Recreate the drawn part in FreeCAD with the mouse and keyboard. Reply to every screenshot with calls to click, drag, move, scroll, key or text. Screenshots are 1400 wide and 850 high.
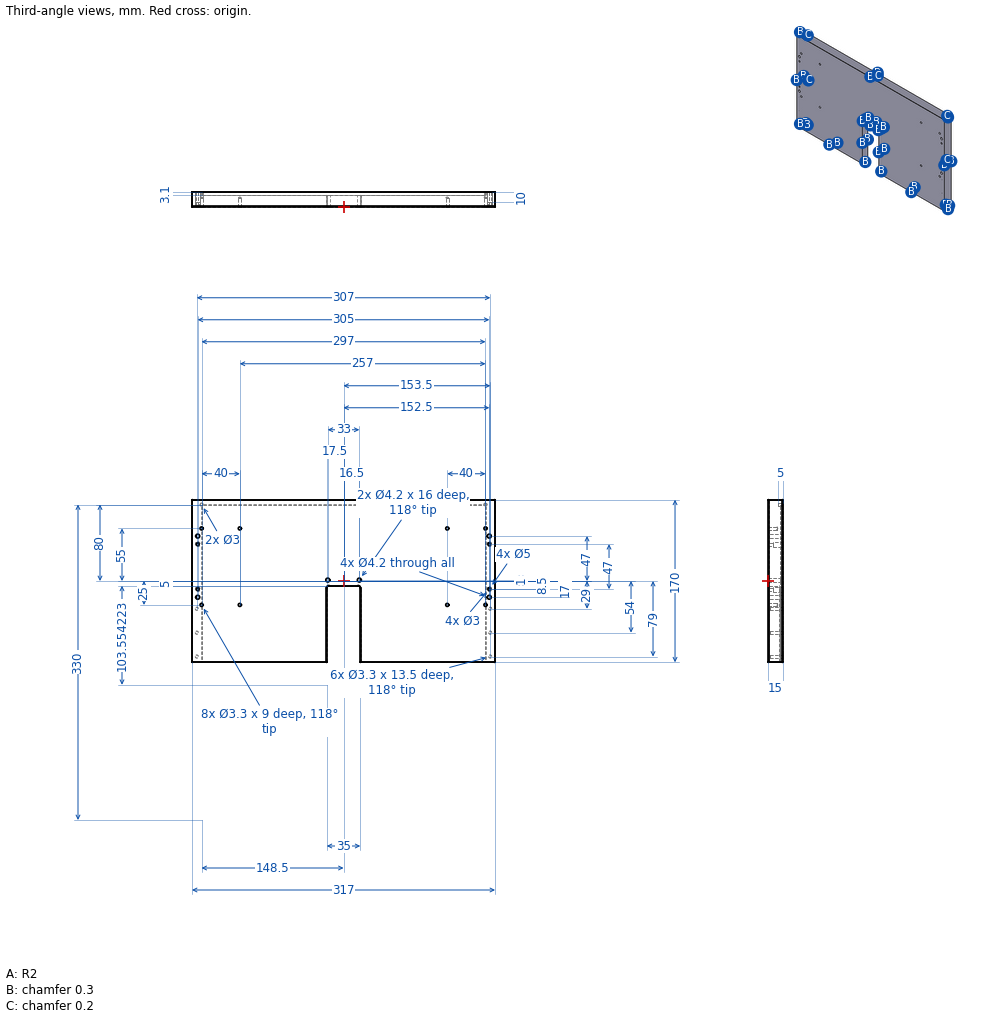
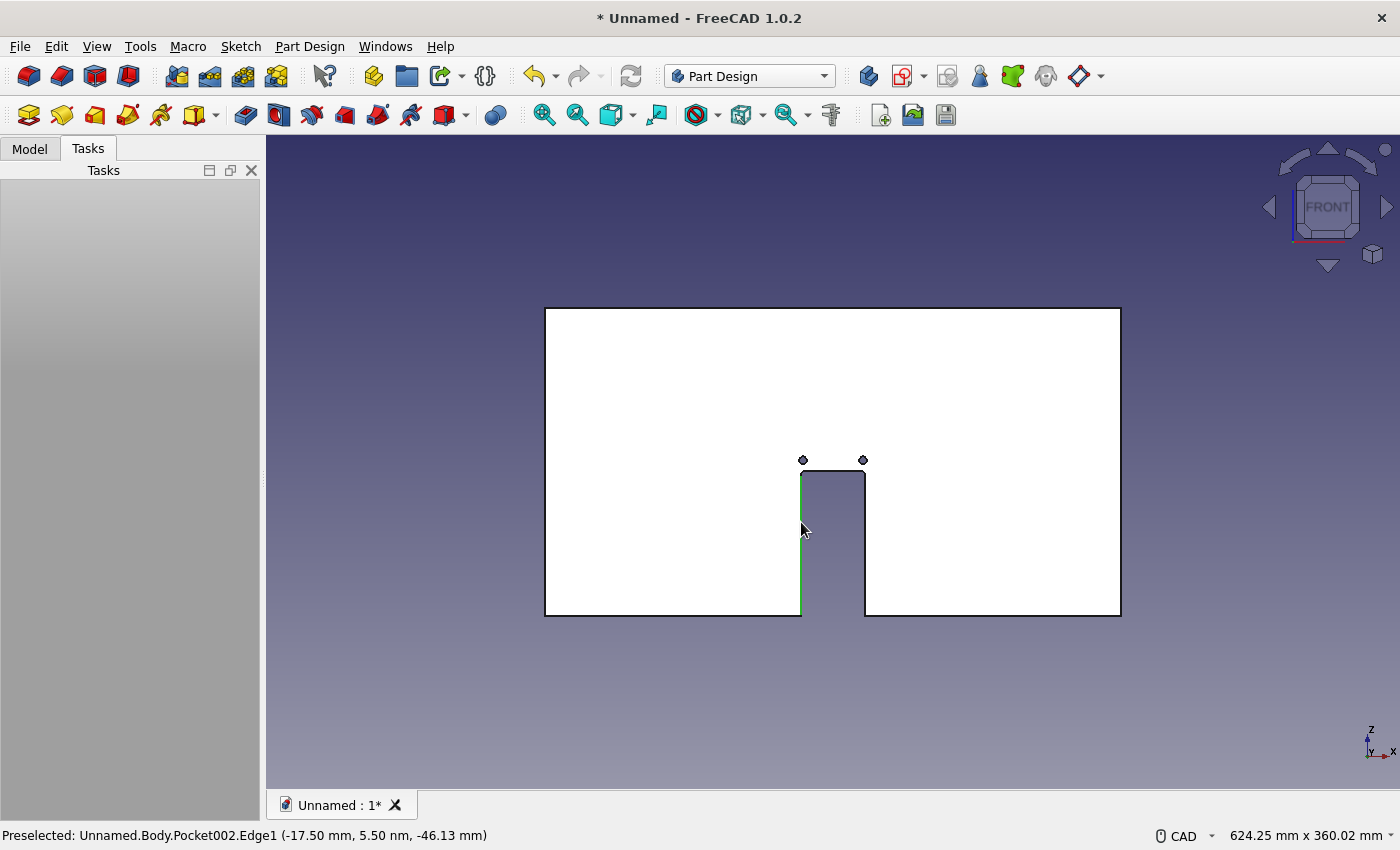
click(865, 545, ctrl)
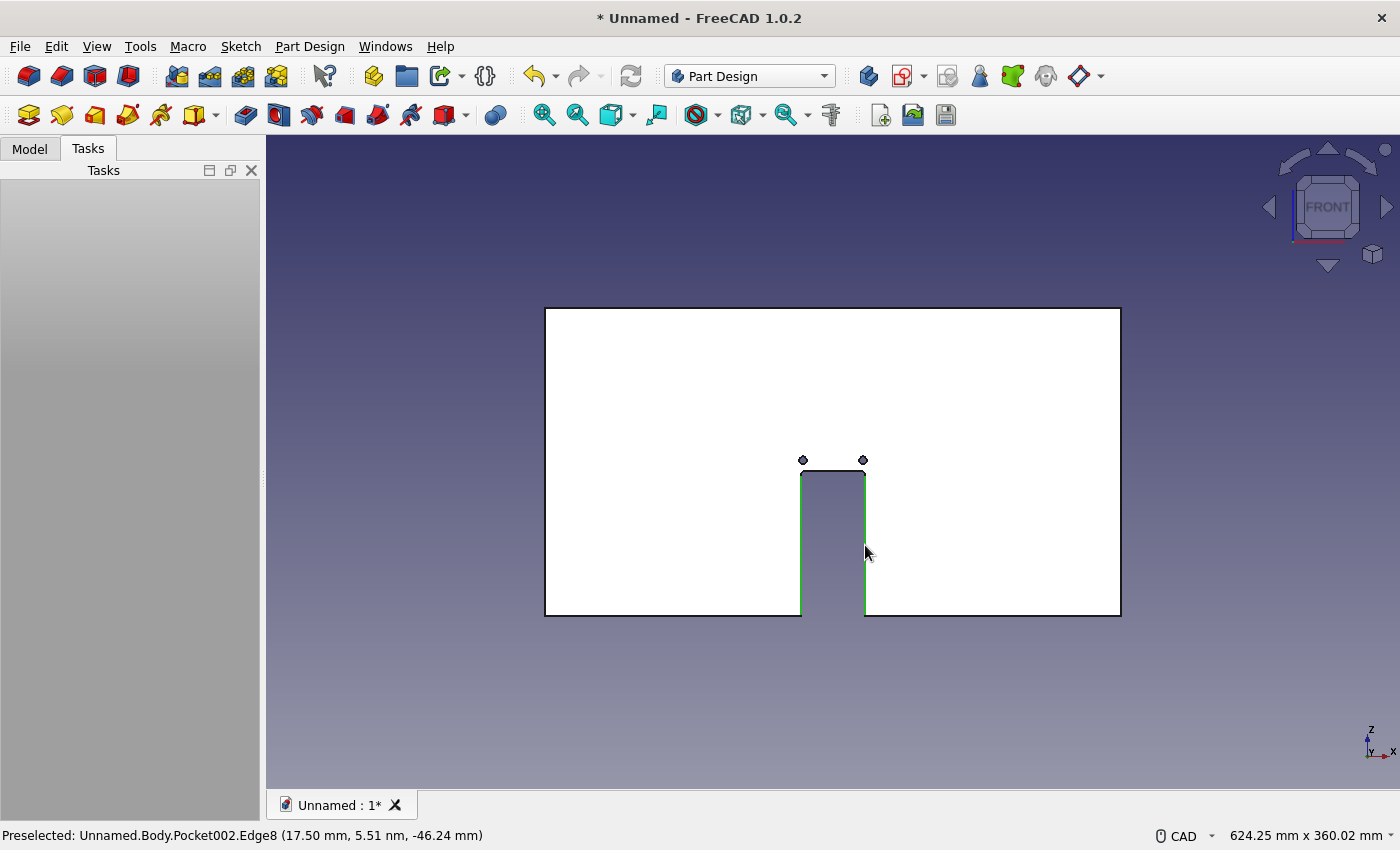
key(3)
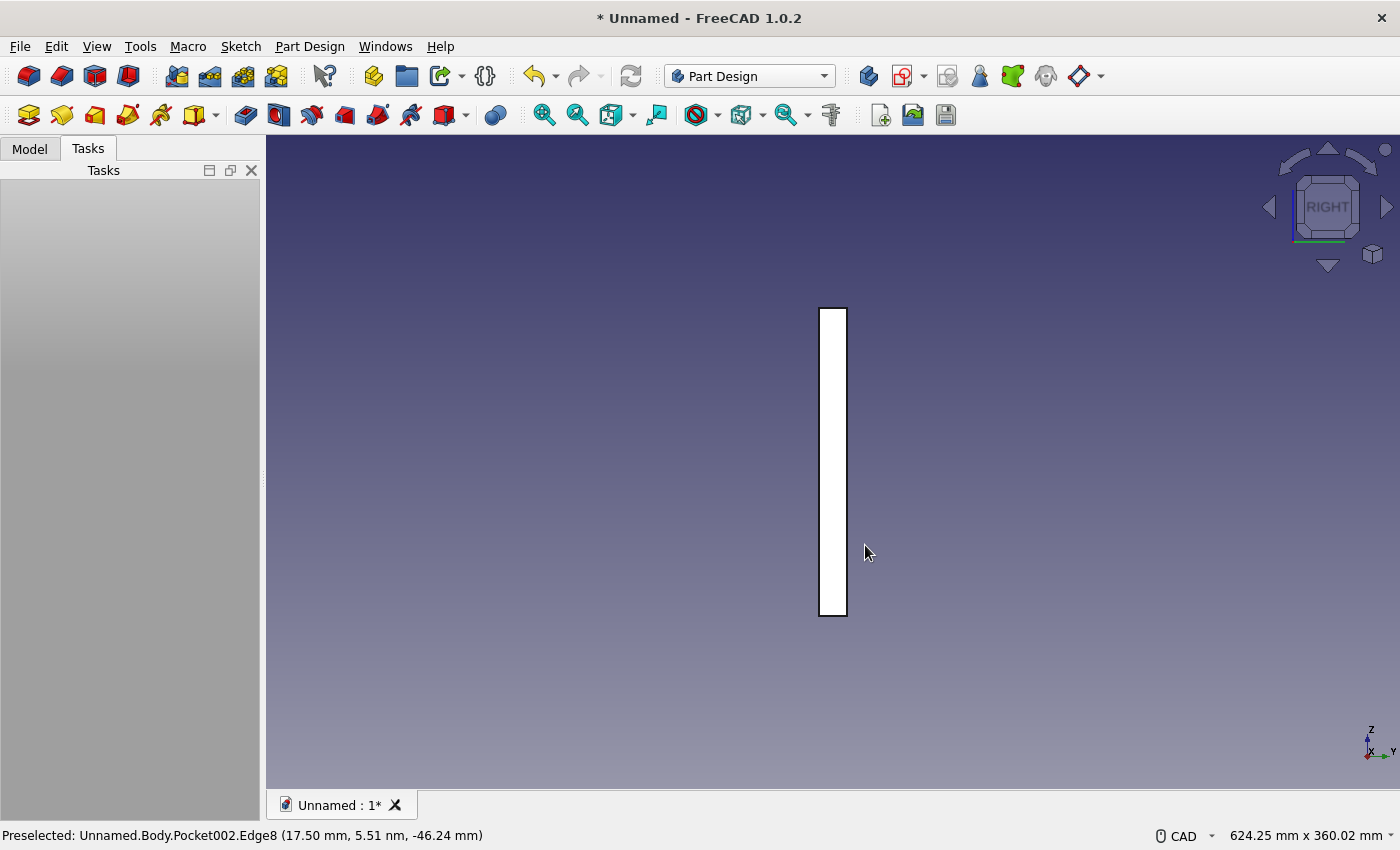
key(5)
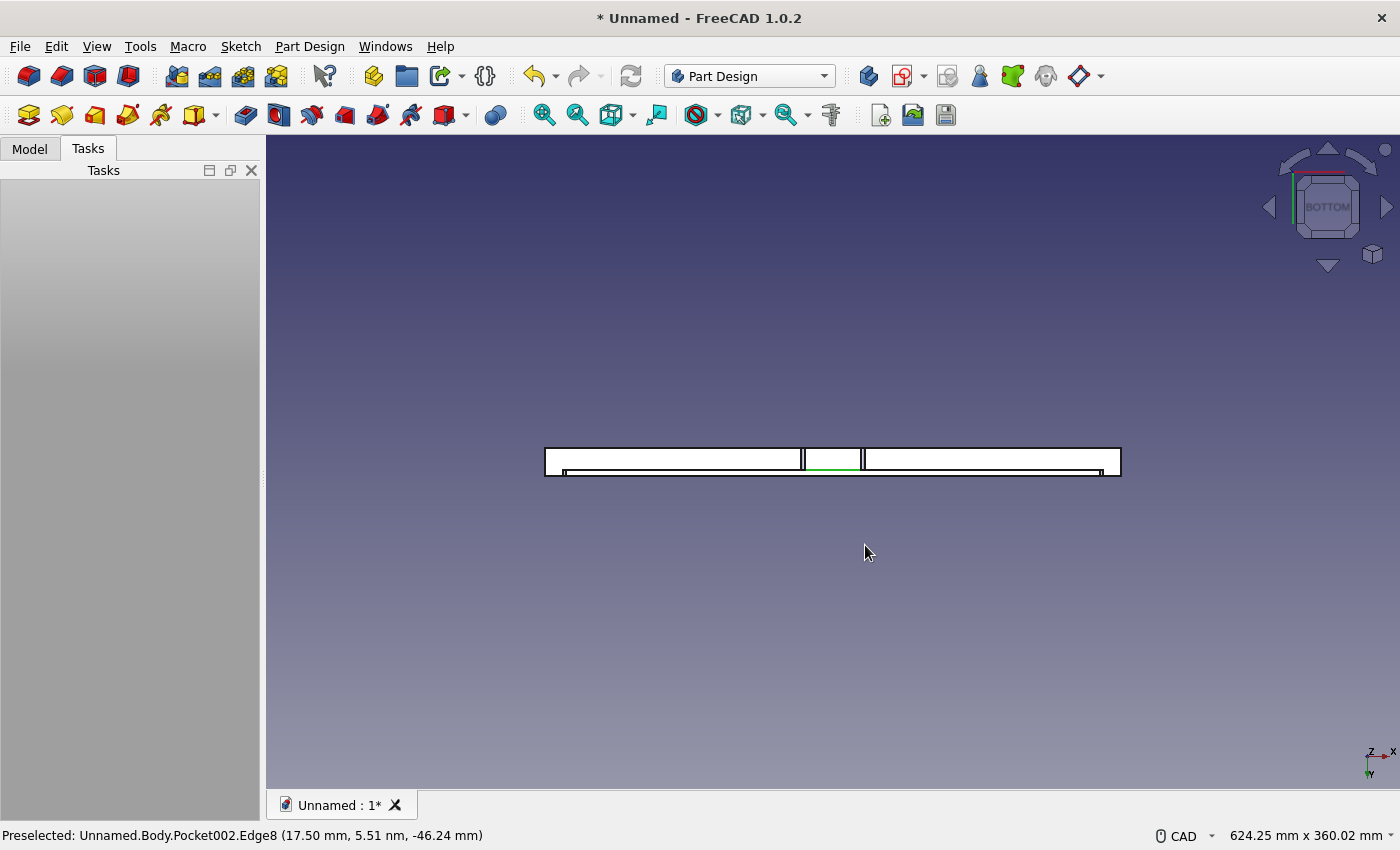
click(783, 457, ctrl)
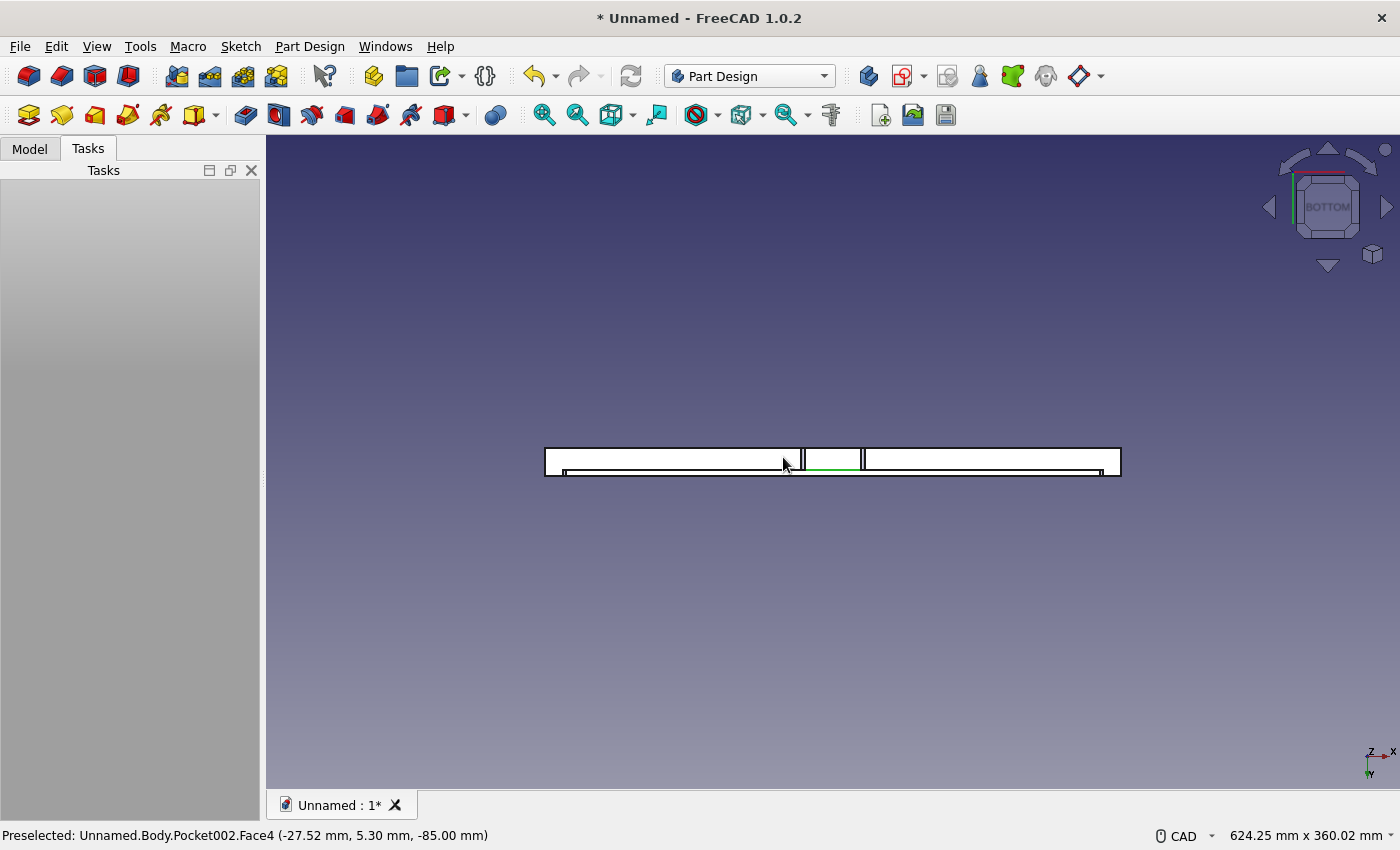
click(1103, 457, ctrl)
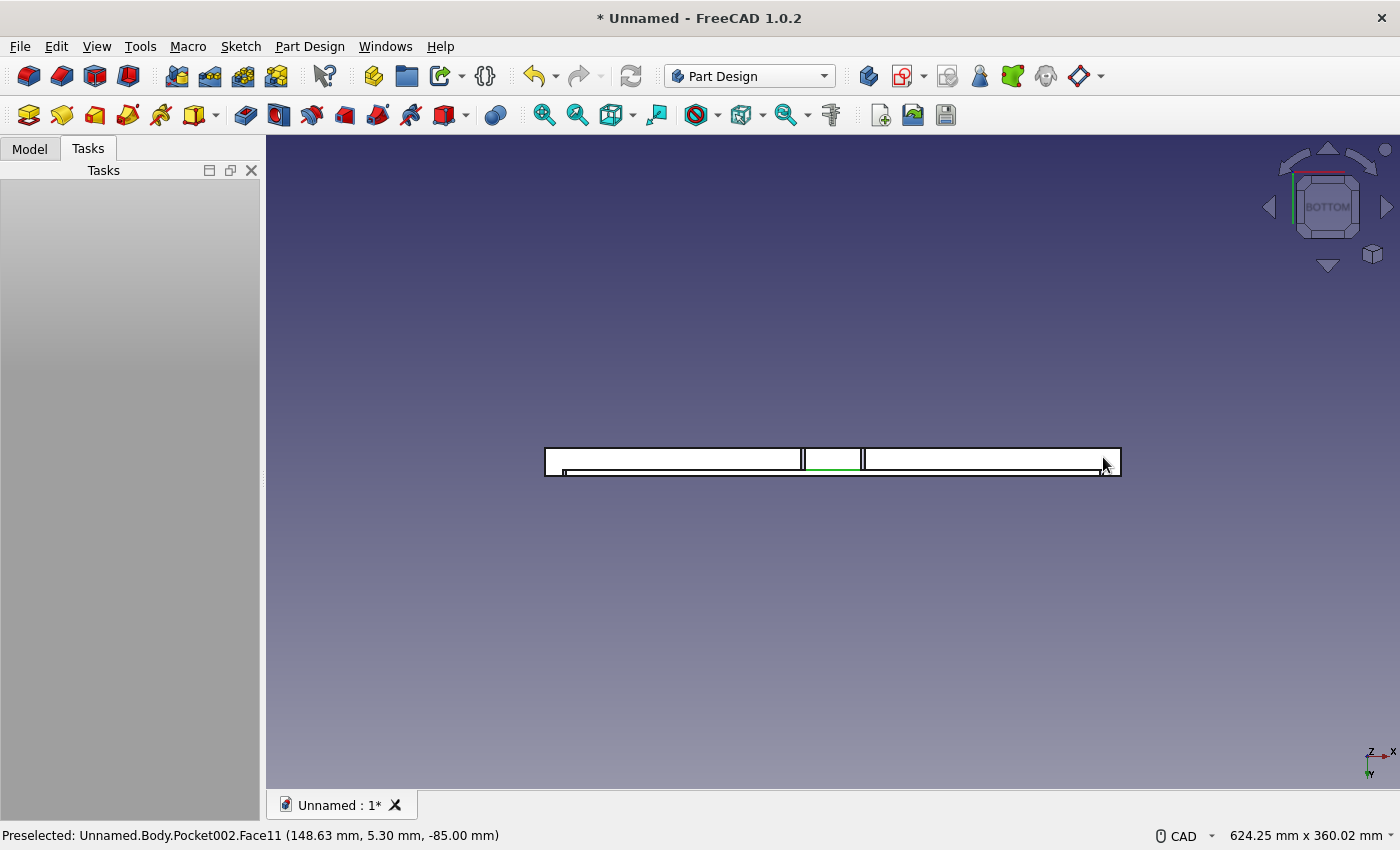
click(833, 447, ctrl)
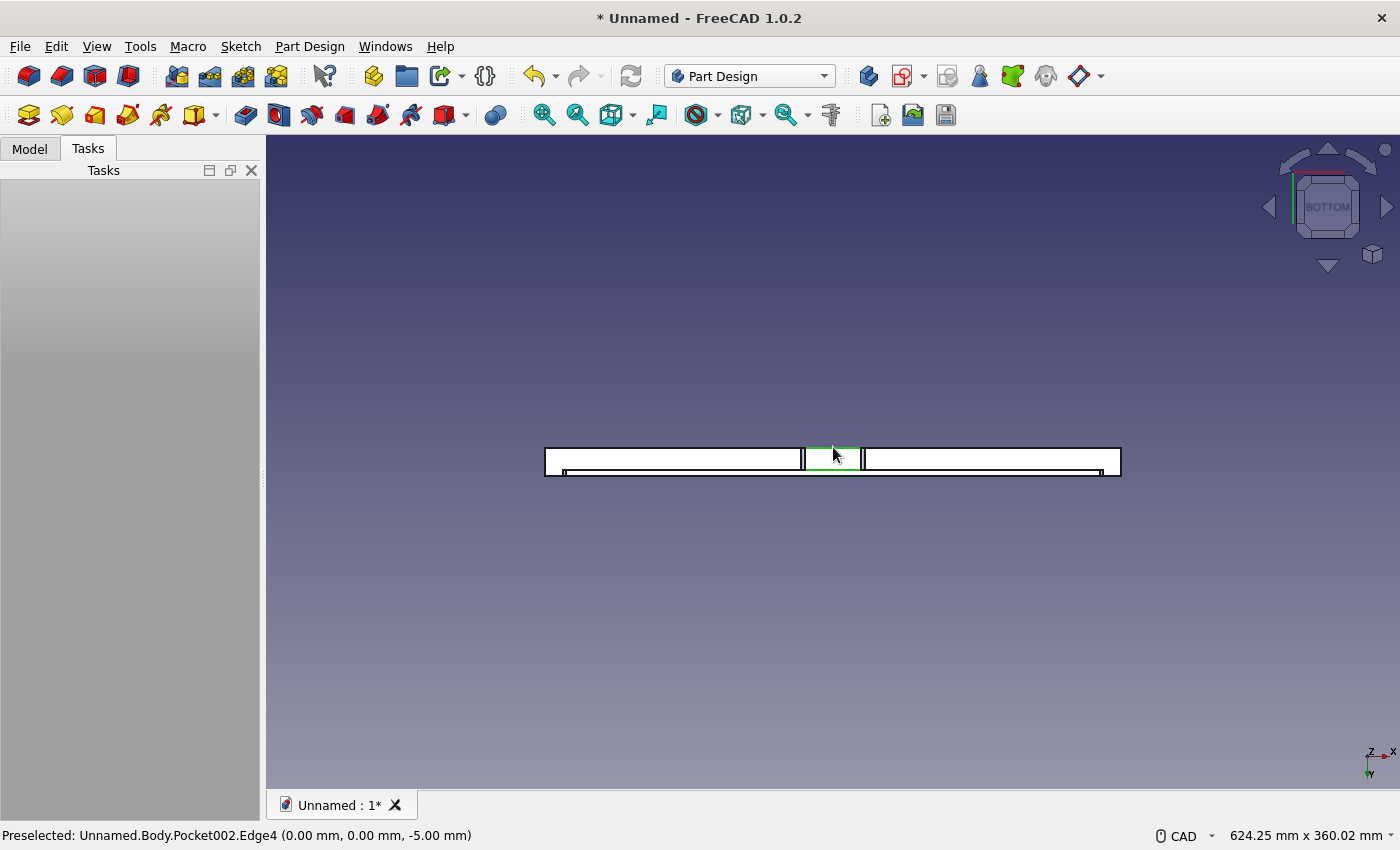
key(4)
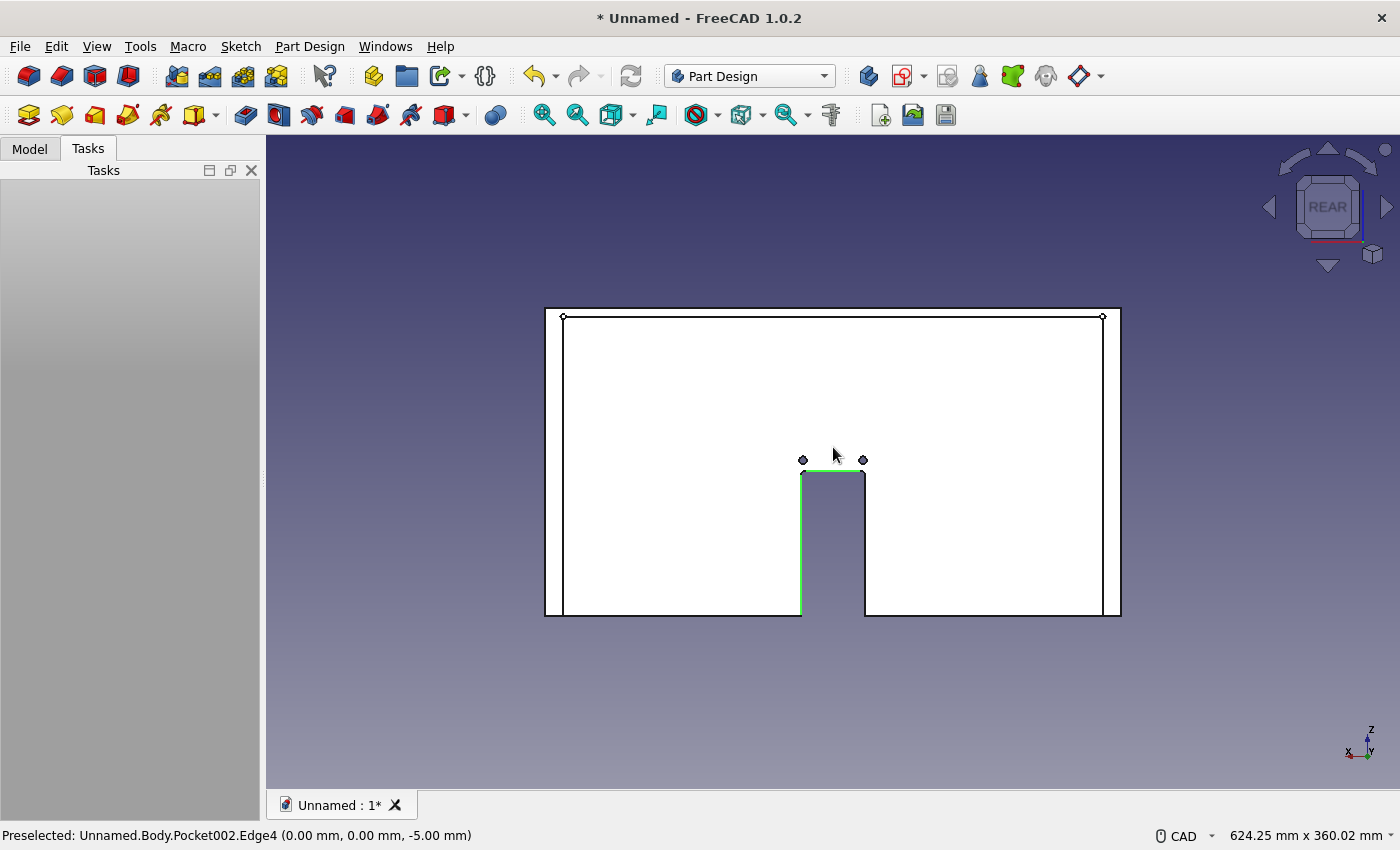
click(865, 545, ctrl)